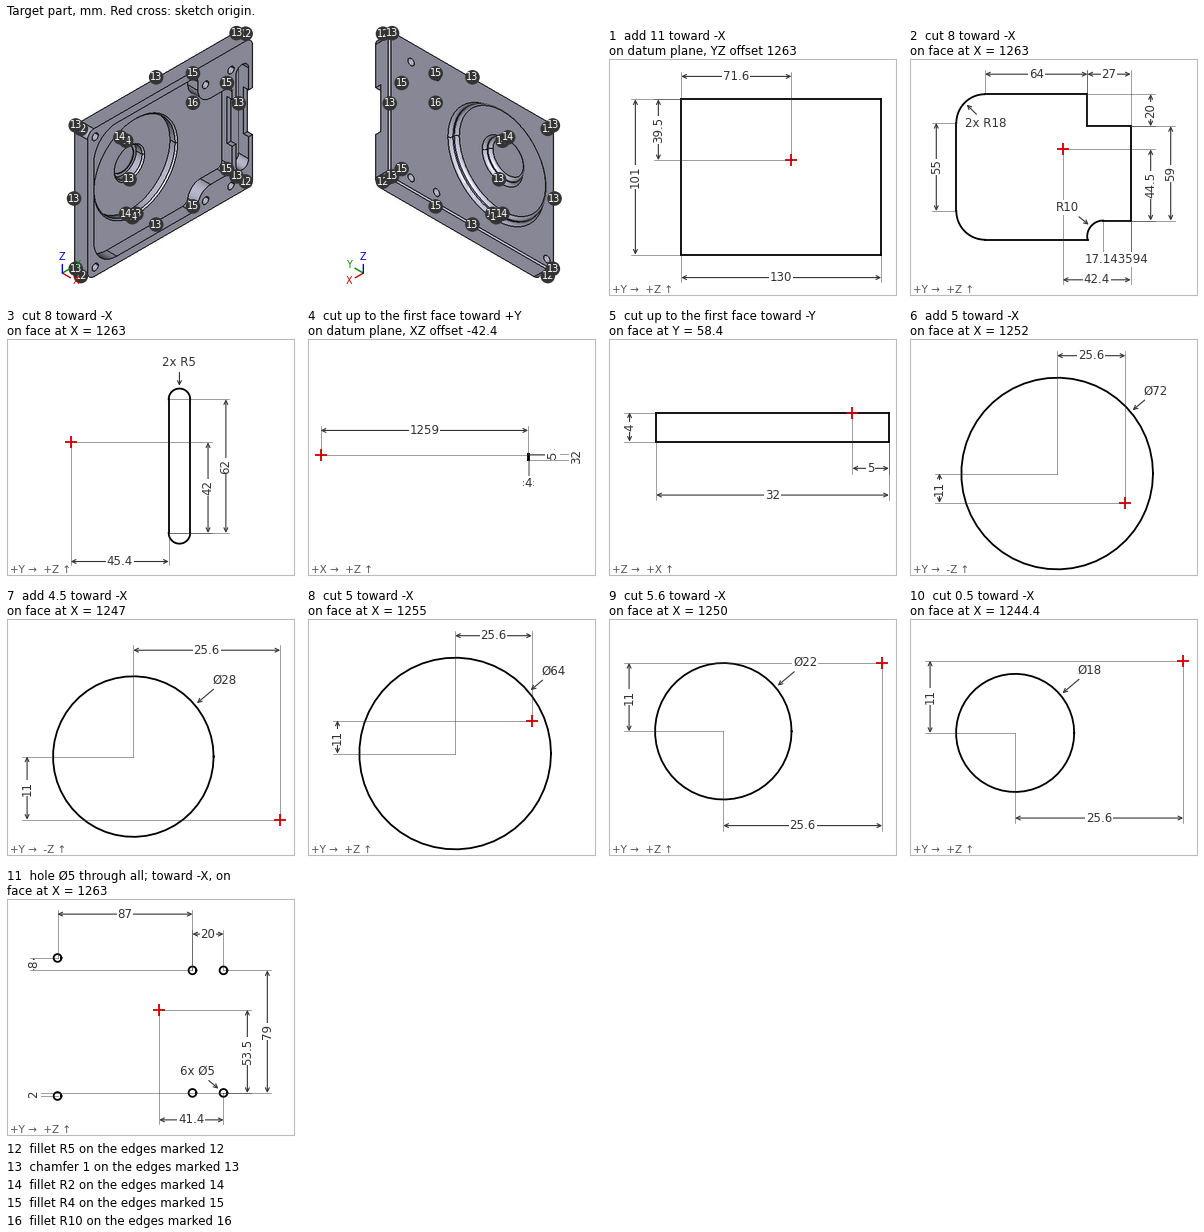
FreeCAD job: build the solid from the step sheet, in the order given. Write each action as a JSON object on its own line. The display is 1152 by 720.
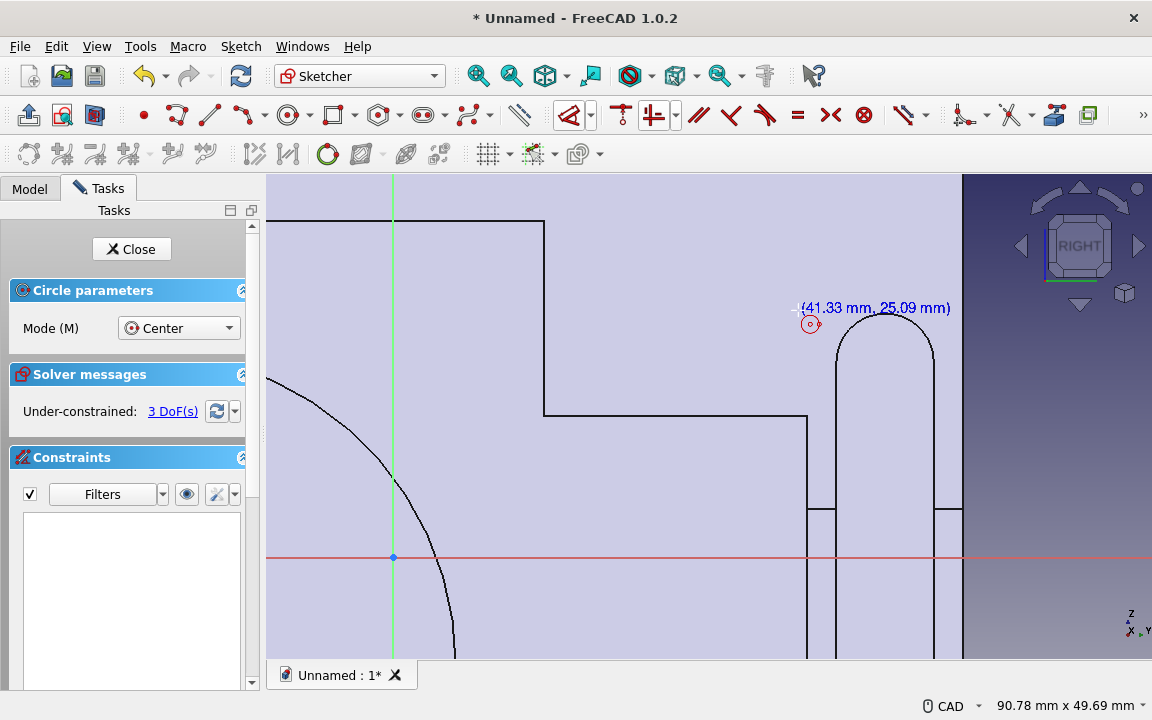
{"action": "left_click", "coordinate": [797, 309]}
{"action": "left_click", "coordinate": [815, 291]}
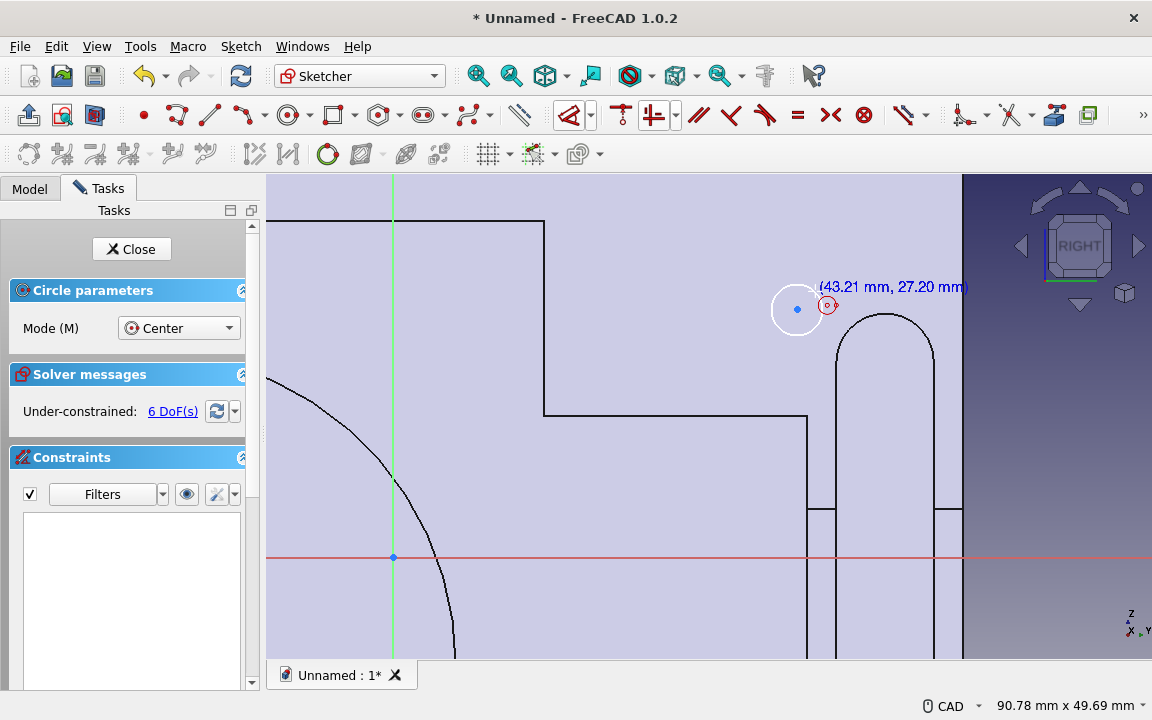
{"action": "left_click", "coordinate": [602, 309]}
{"action": "left_click", "coordinate": [619, 291]}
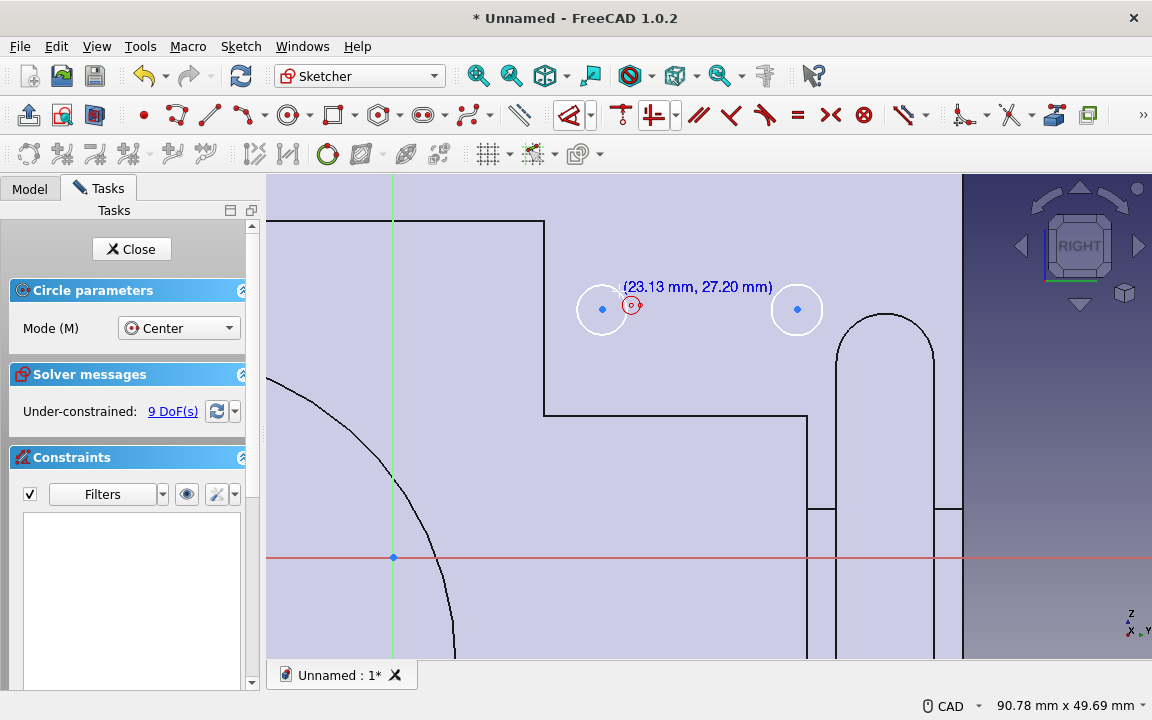
{"action": "scroll", "coordinate": [798, 309], "scroll_direction": "down", "scroll_amount": 6}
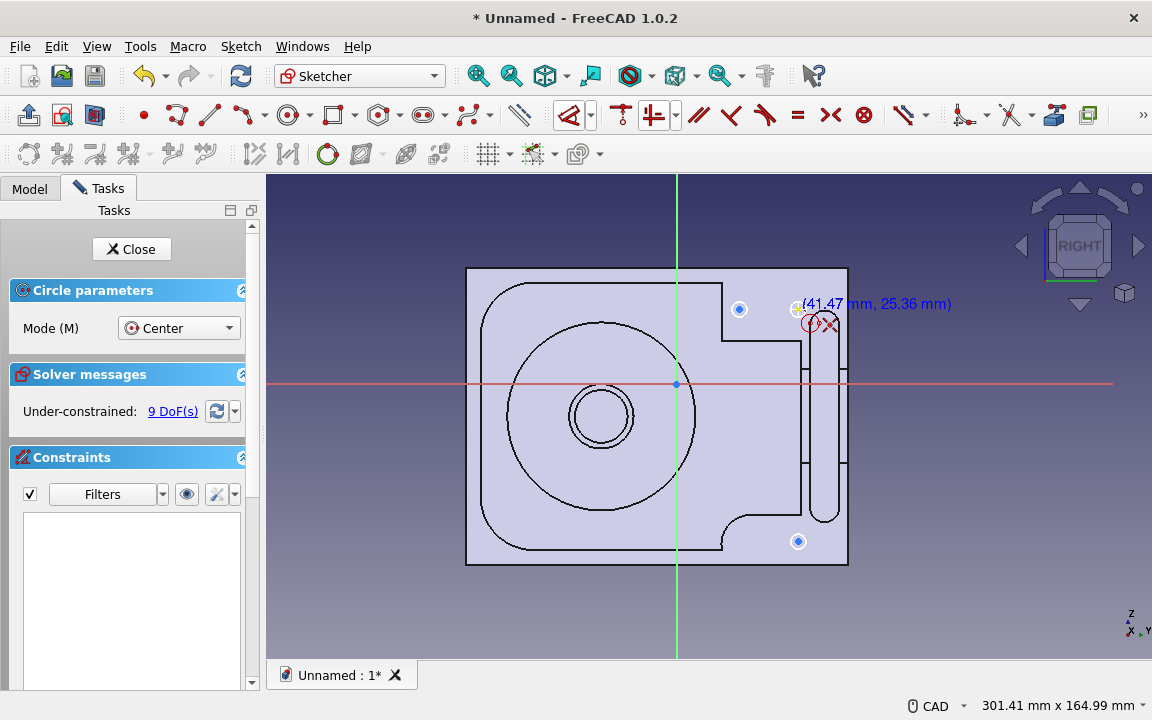
{"action": "scroll", "coordinate": [484, 286], "scroll_direction": "up", "scroll_amount": 6}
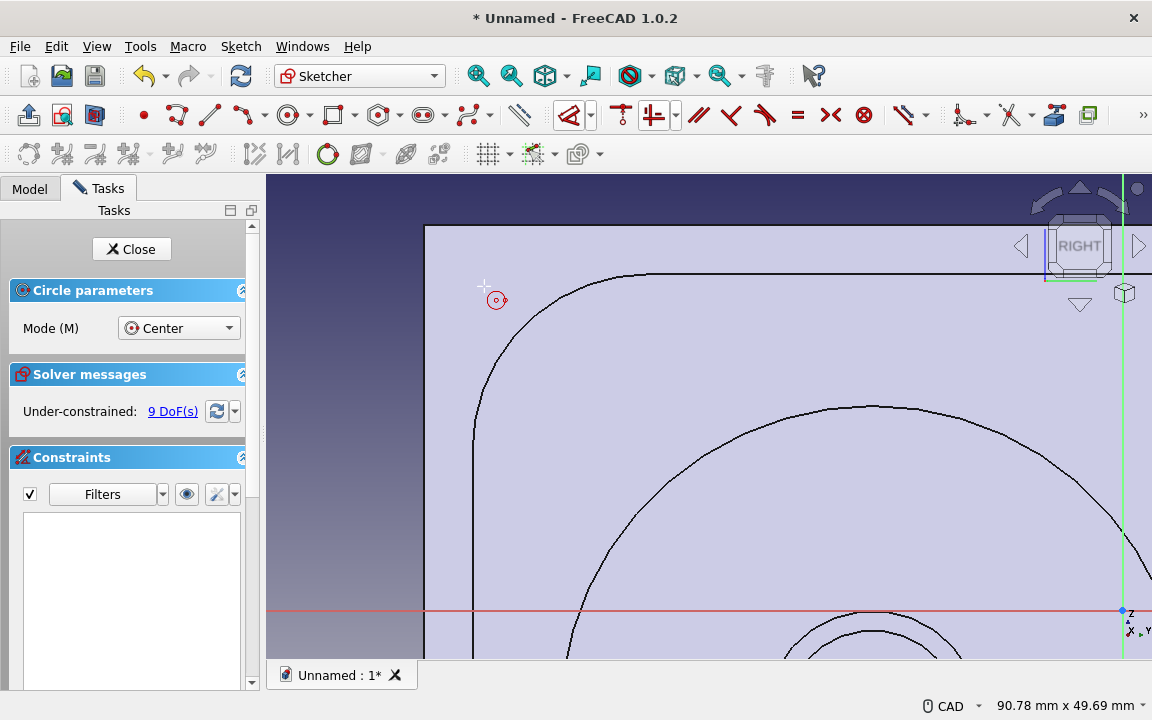
{"action": "left_click", "coordinate": [482, 284]}
{"action": "left_click", "coordinate": [500, 267]}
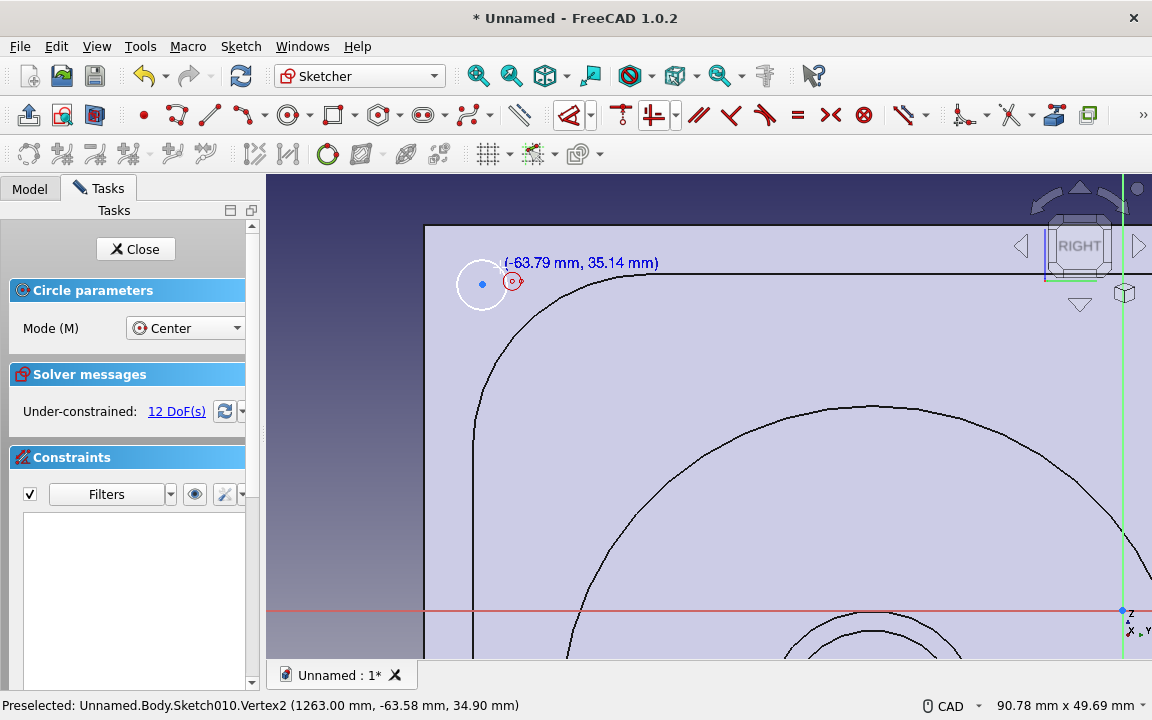
{"action": "scroll", "coordinate": [484, 286], "scroll_direction": "down", "scroll_amount": 6}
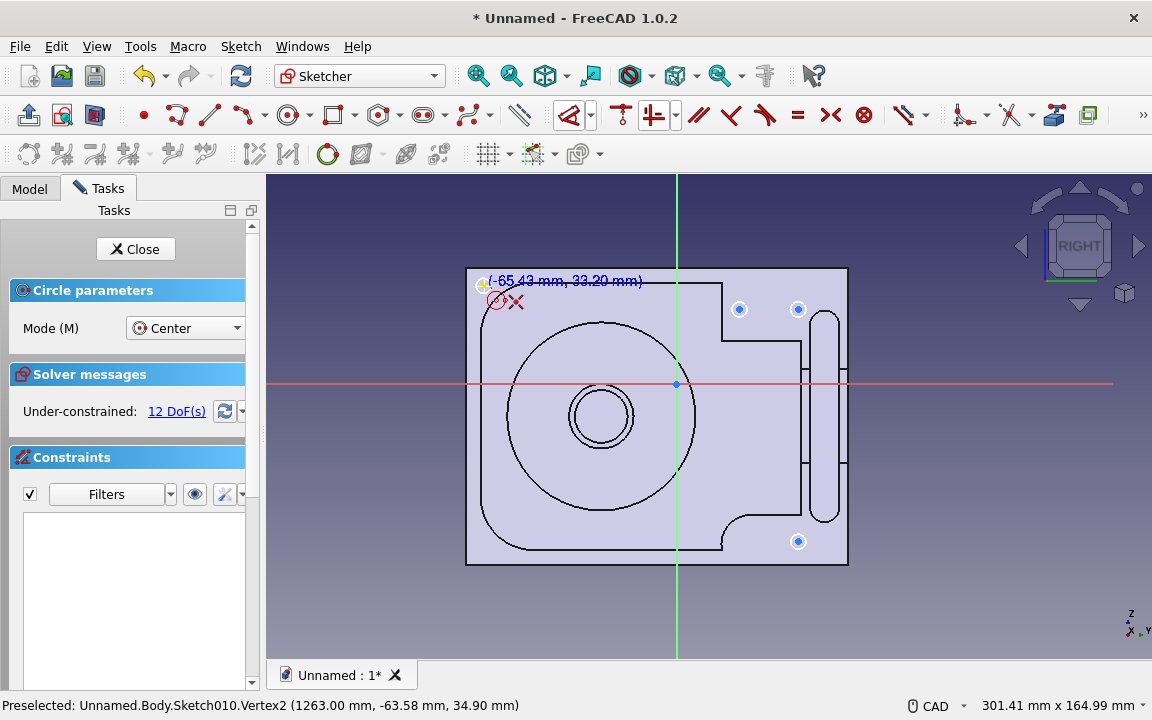
{"action": "scroll", "coordinate": [484, 547], "scroll_direction": "up", "scroll_amount": 6}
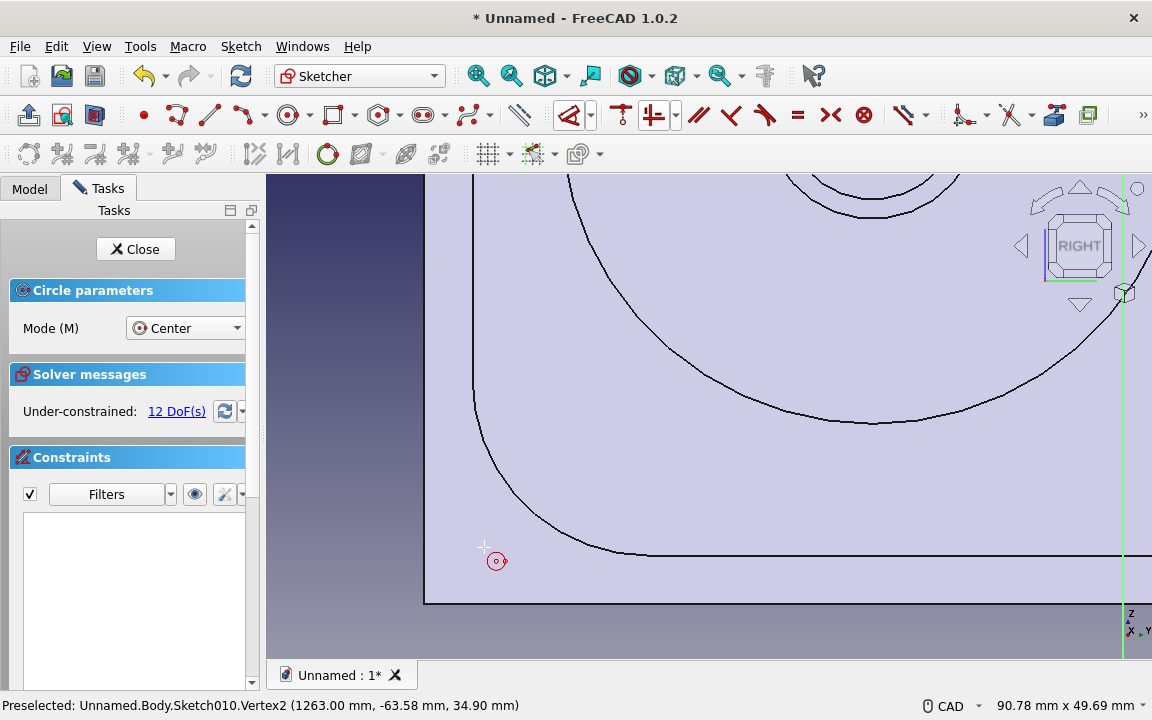
{"action": "left_click", "coordinate": [482, 546]}
{"action": "left_click", "coordinate": [500, 529]}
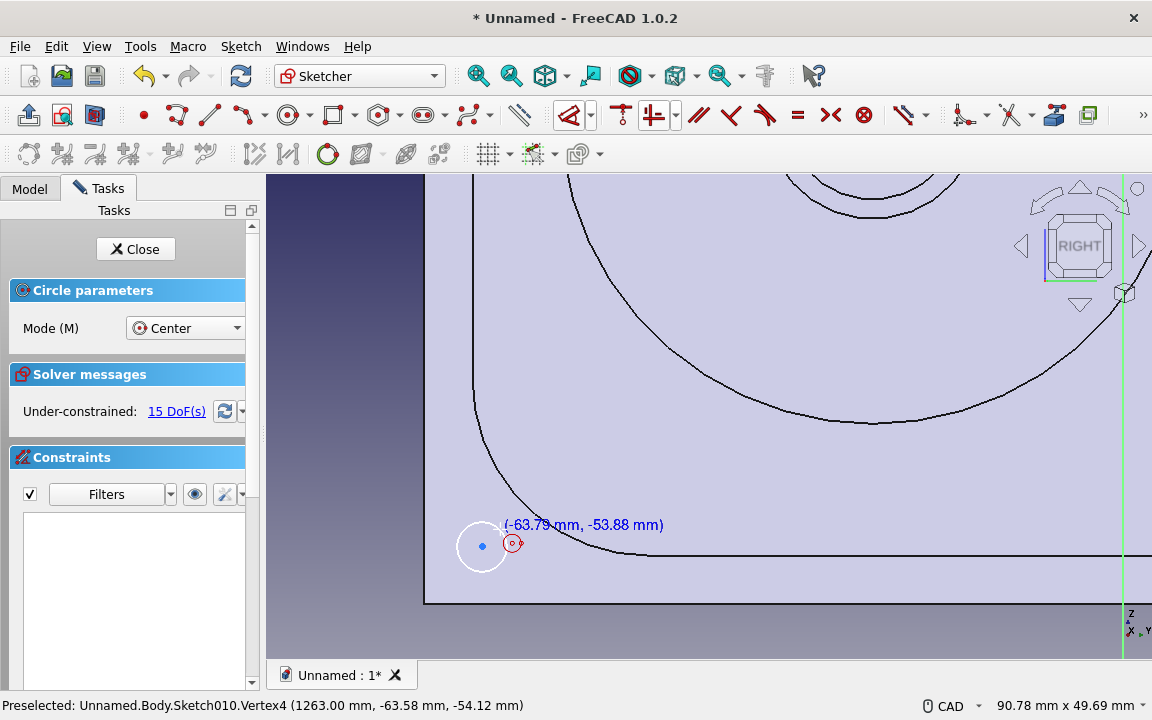
{"action": "scroll", "coordinate": [484, 548], "scroll_direction": "down", "scroll_amount": 6}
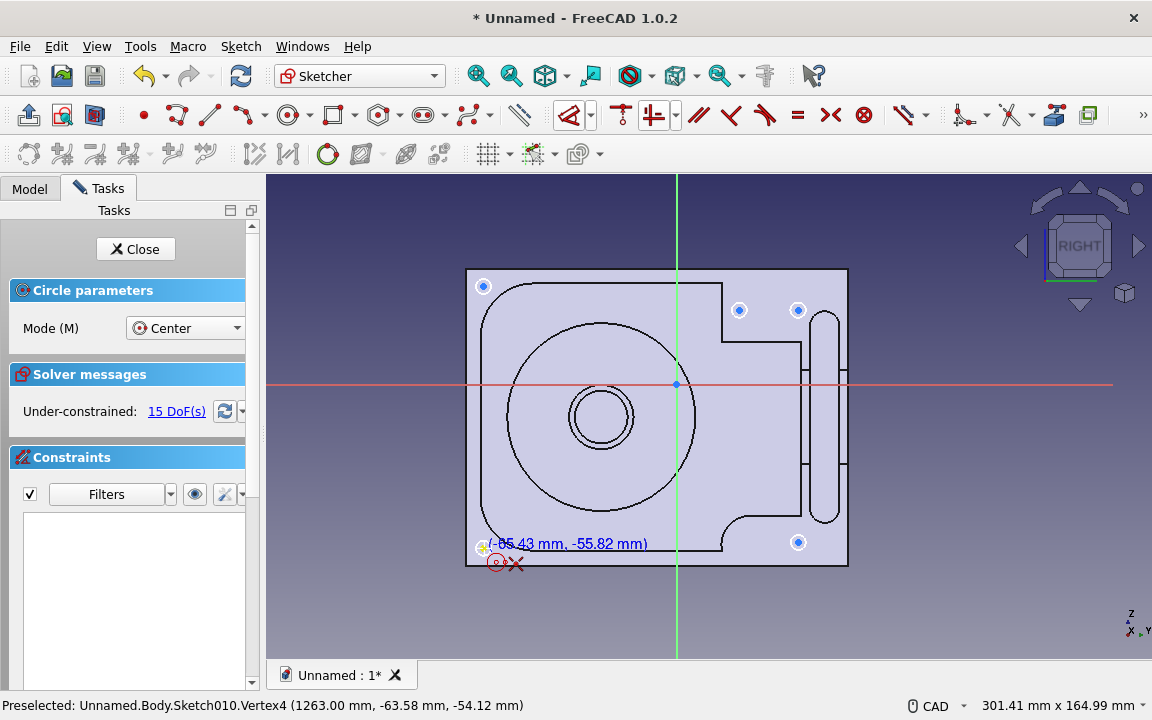
{"action": "scroll", "coordinate": [739, 542], "scroll_direction": "up", "scroll_amount": 6}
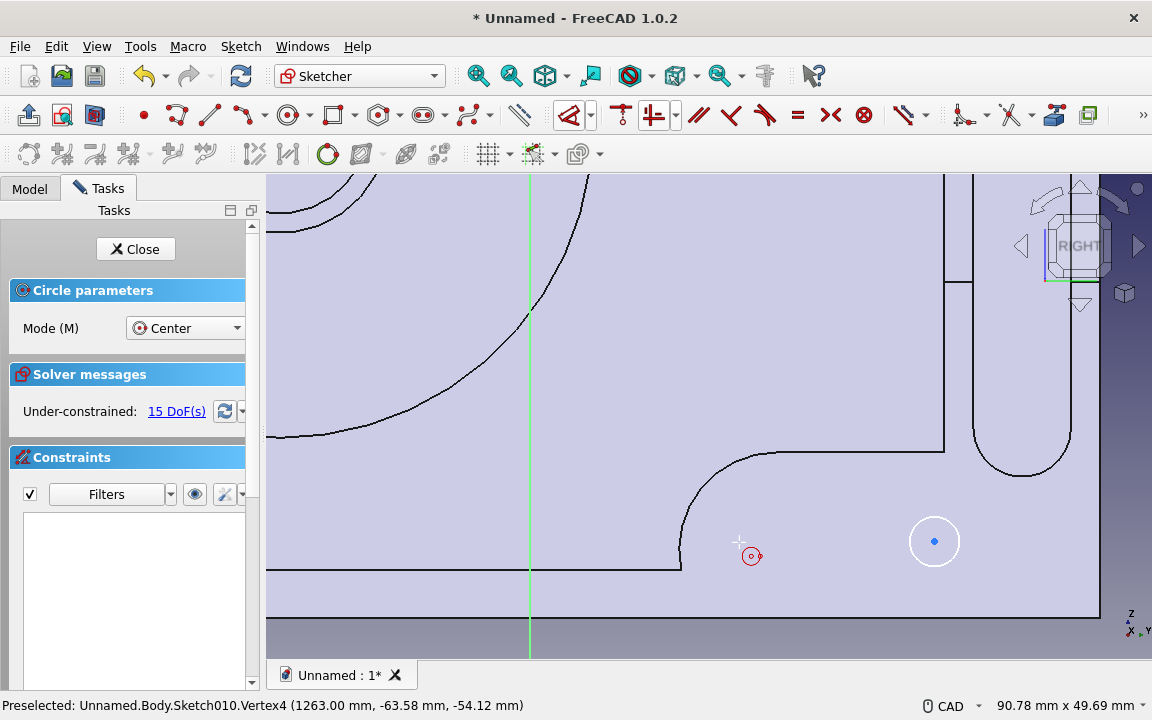
{"action": "left_click", "coordinate": [739, 540]}
{"action": "left_click", "coordinate": [756, 523]}
{"action": "key", "text": "Escape"}